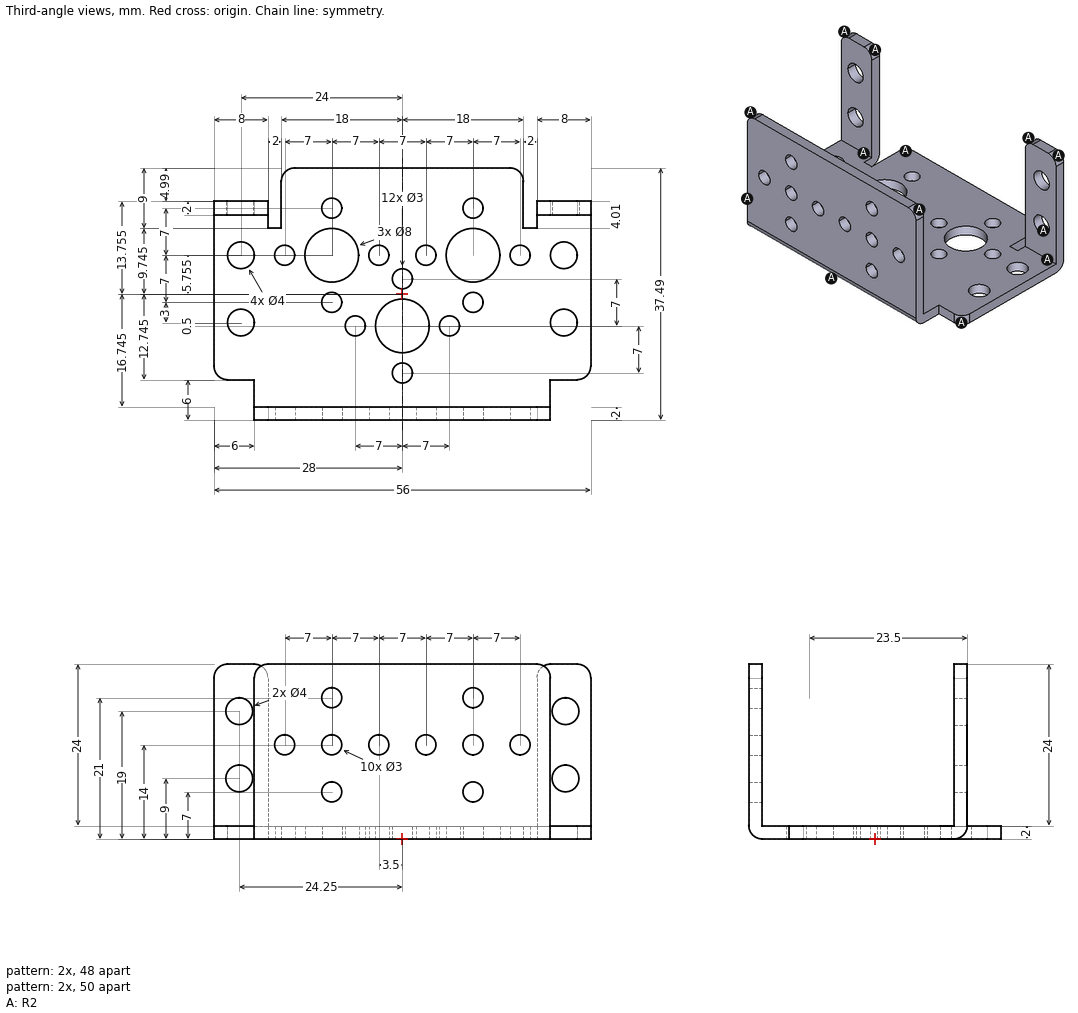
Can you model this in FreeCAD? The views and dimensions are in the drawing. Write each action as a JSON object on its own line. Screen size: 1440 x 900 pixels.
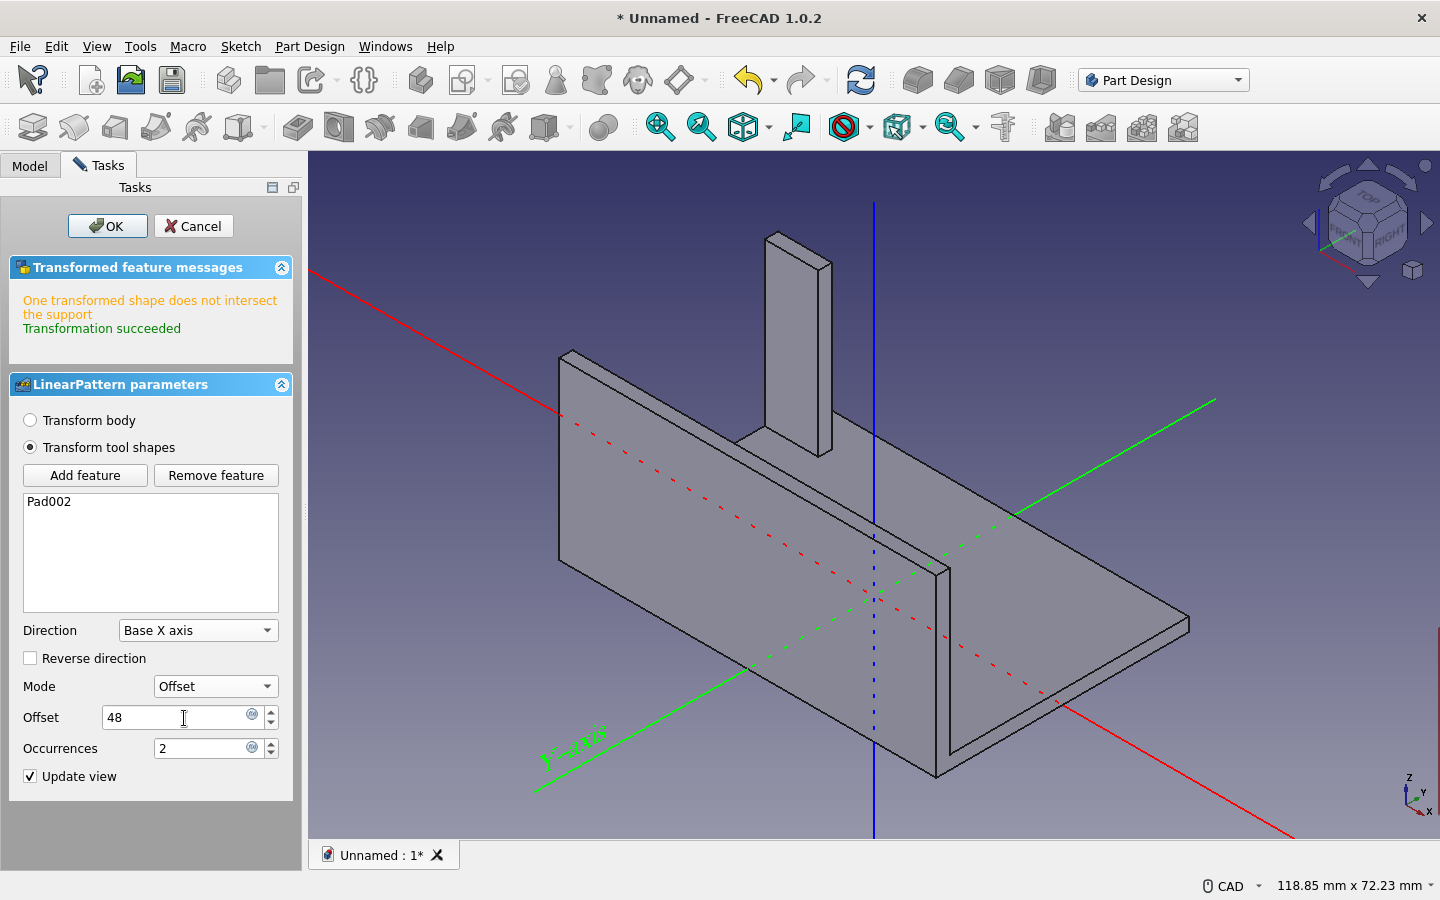
{"action": "triple_click", "coordinate": [210, 748]}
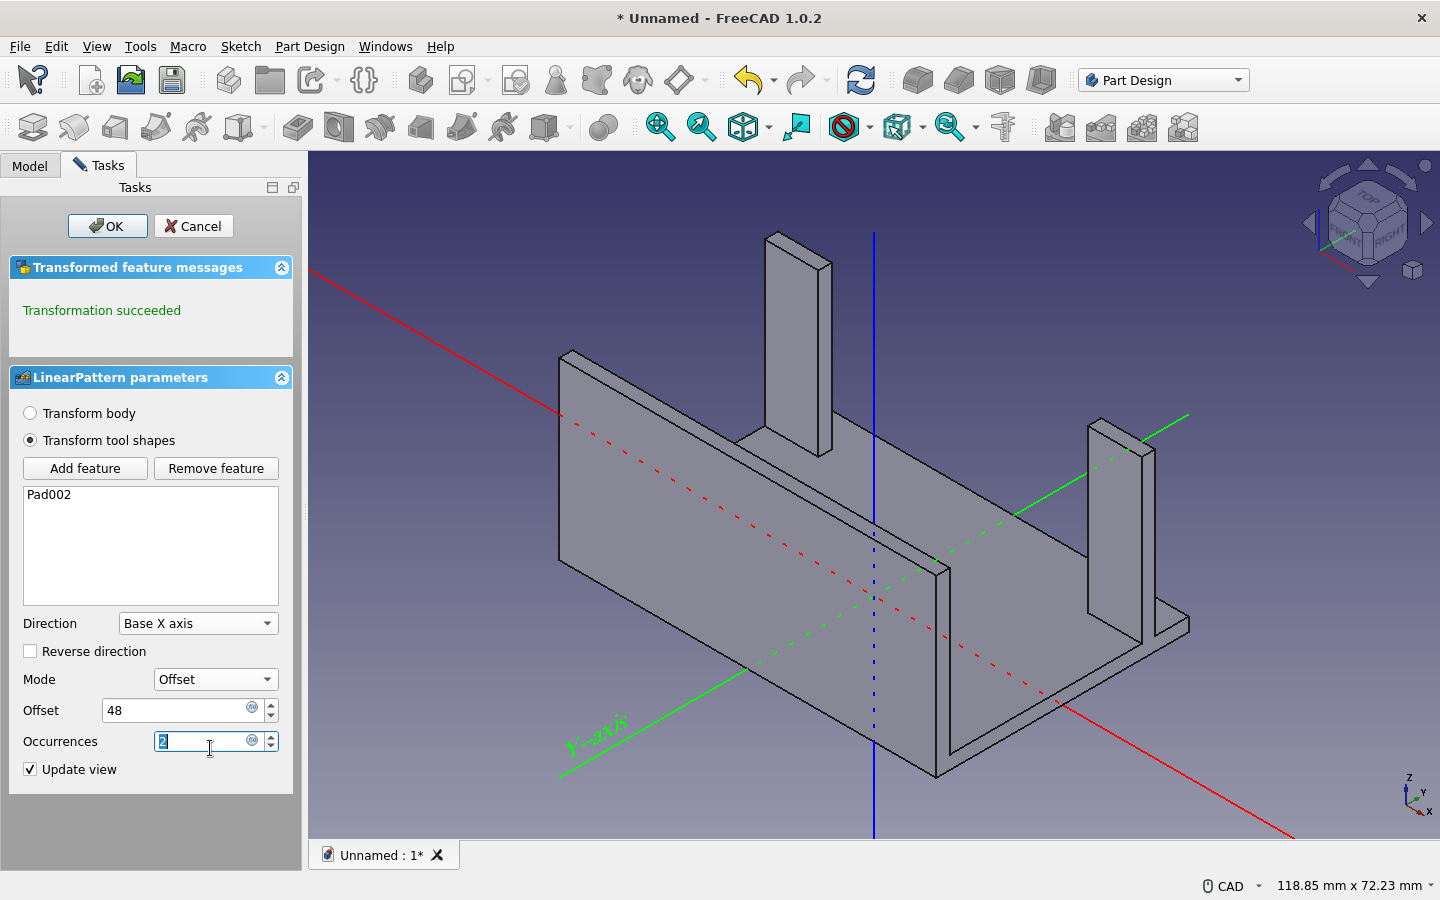
{"action": "type", "text": "2"}
{"action": "key", "text": "Tab"}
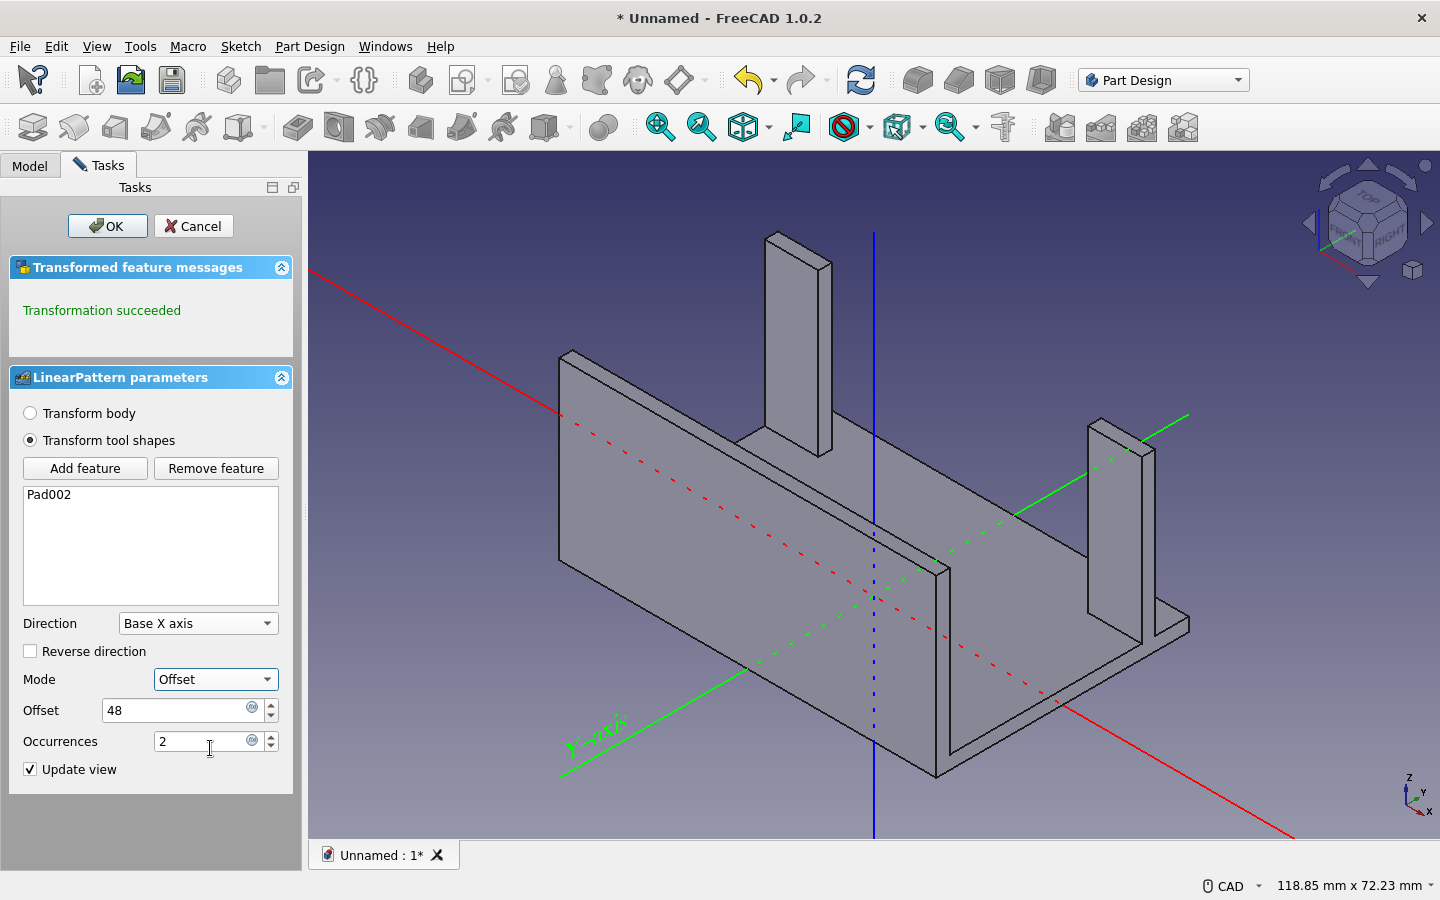
{"action": "left_click", "coordinate": [108, 226]}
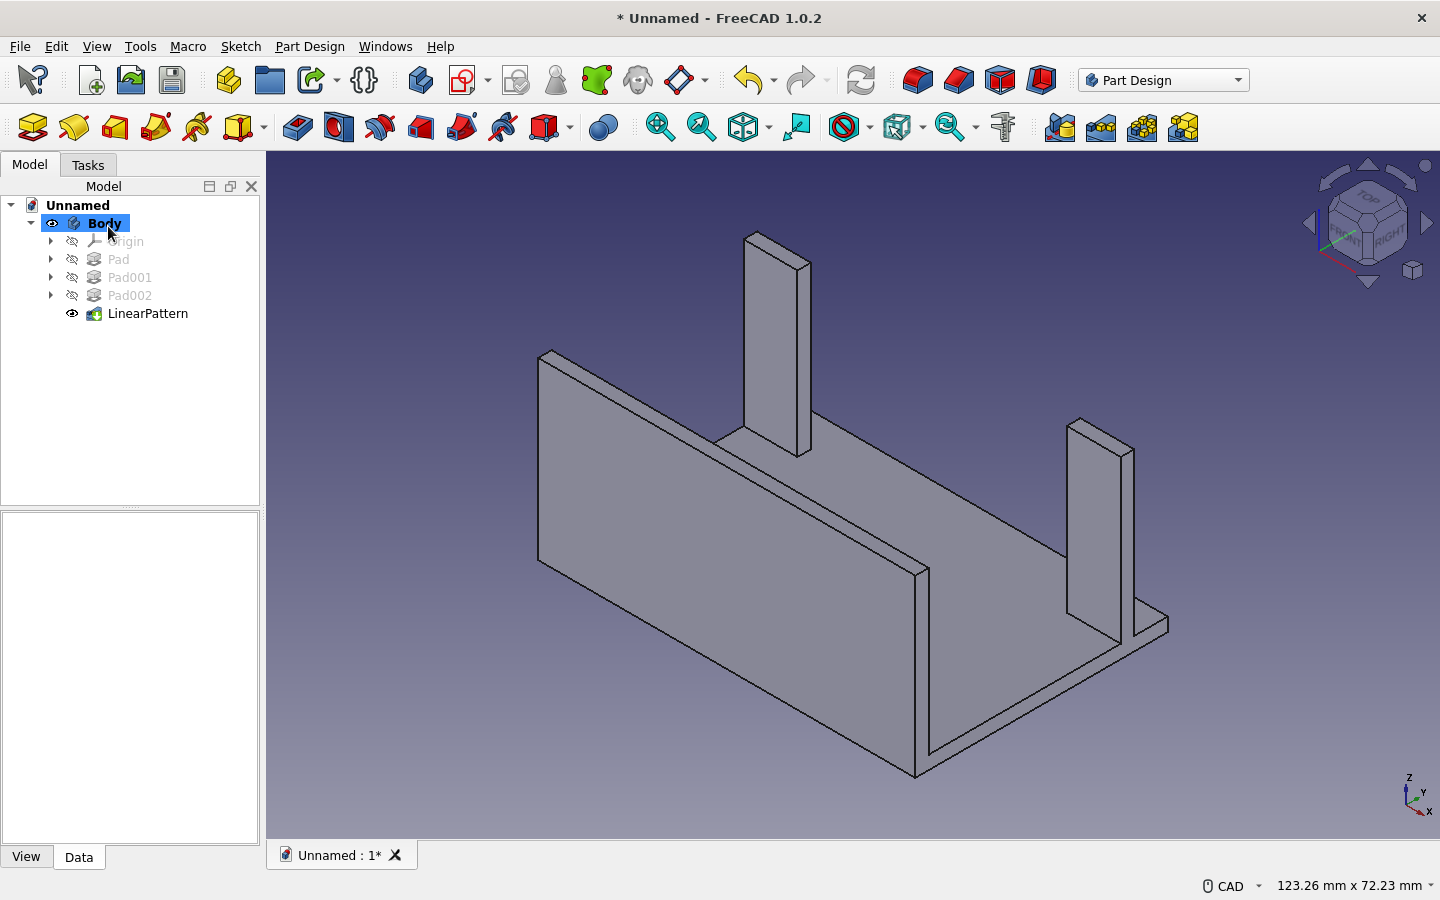
{"action": "left_click", "coordinate": [948, 587]}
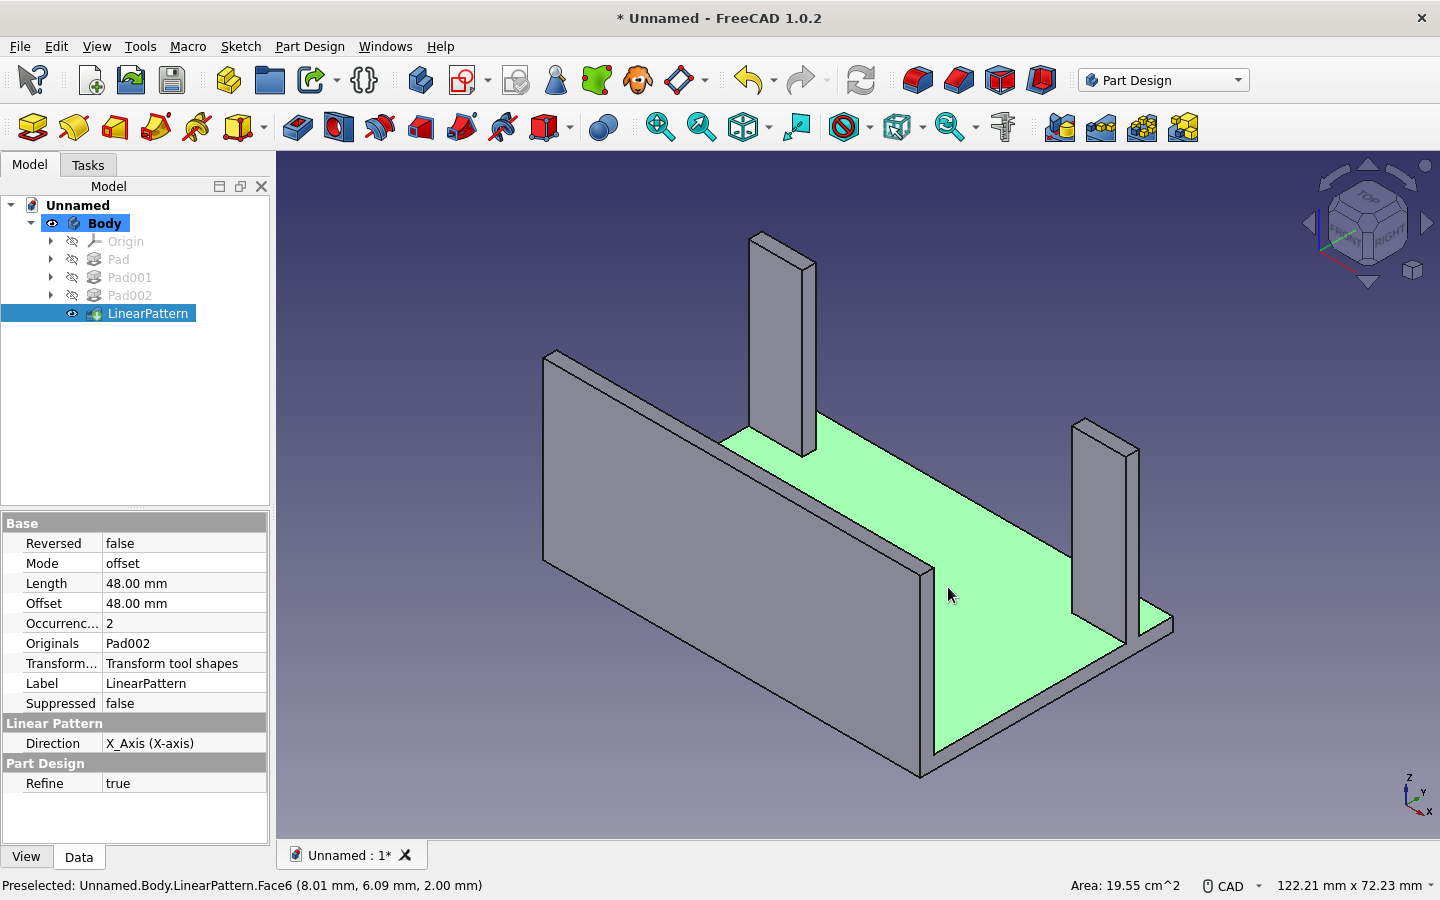
{"action": "left_click", "coordinate": [462, 80]}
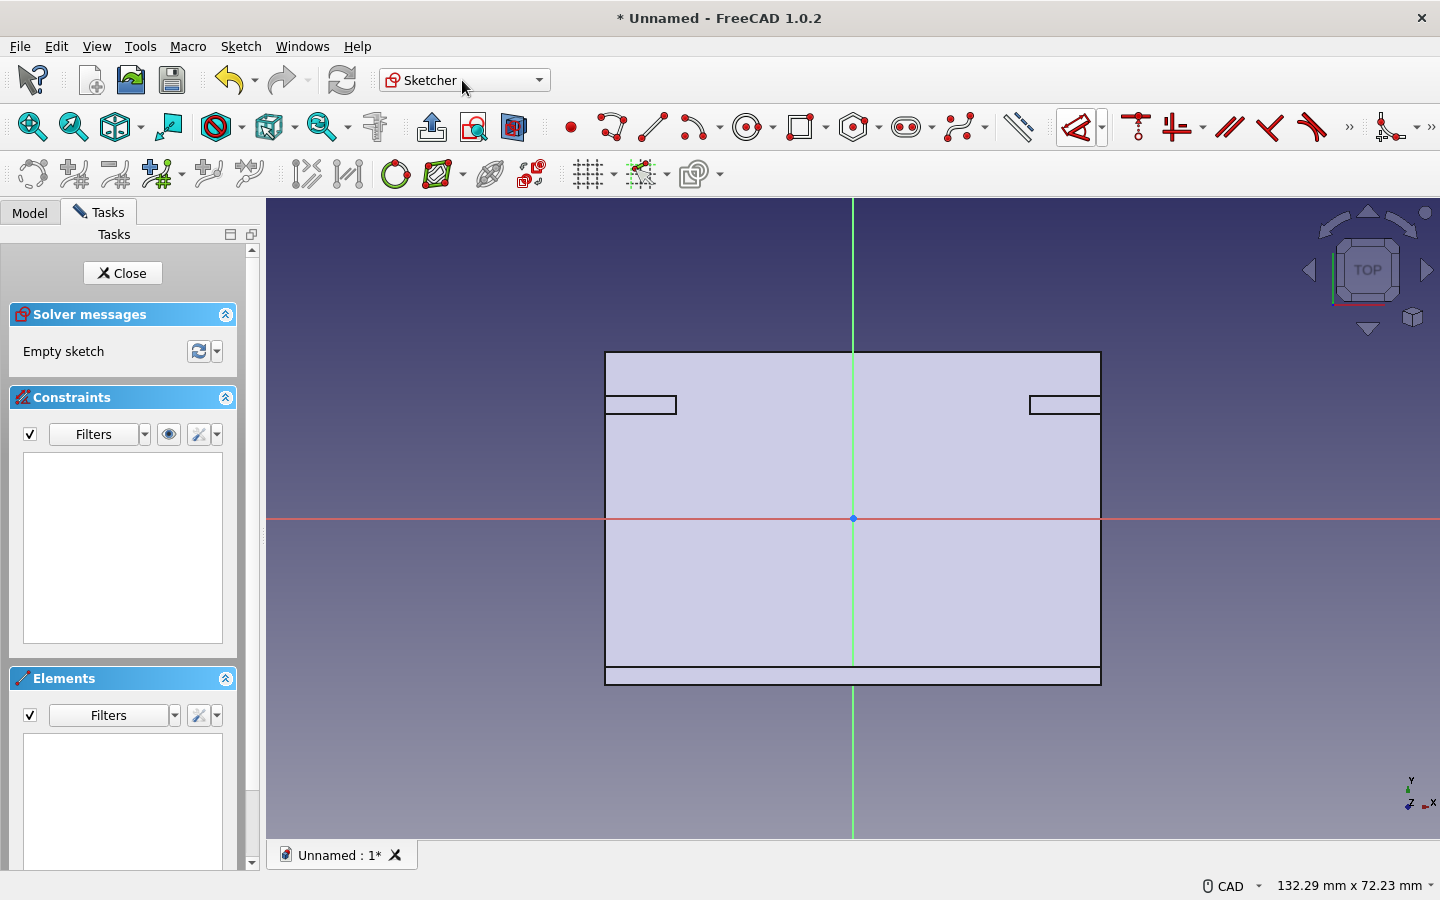
{"action": "scroll", "coordinate": [607, 680], "scroll_direction": "up", "scroll_amount": 10}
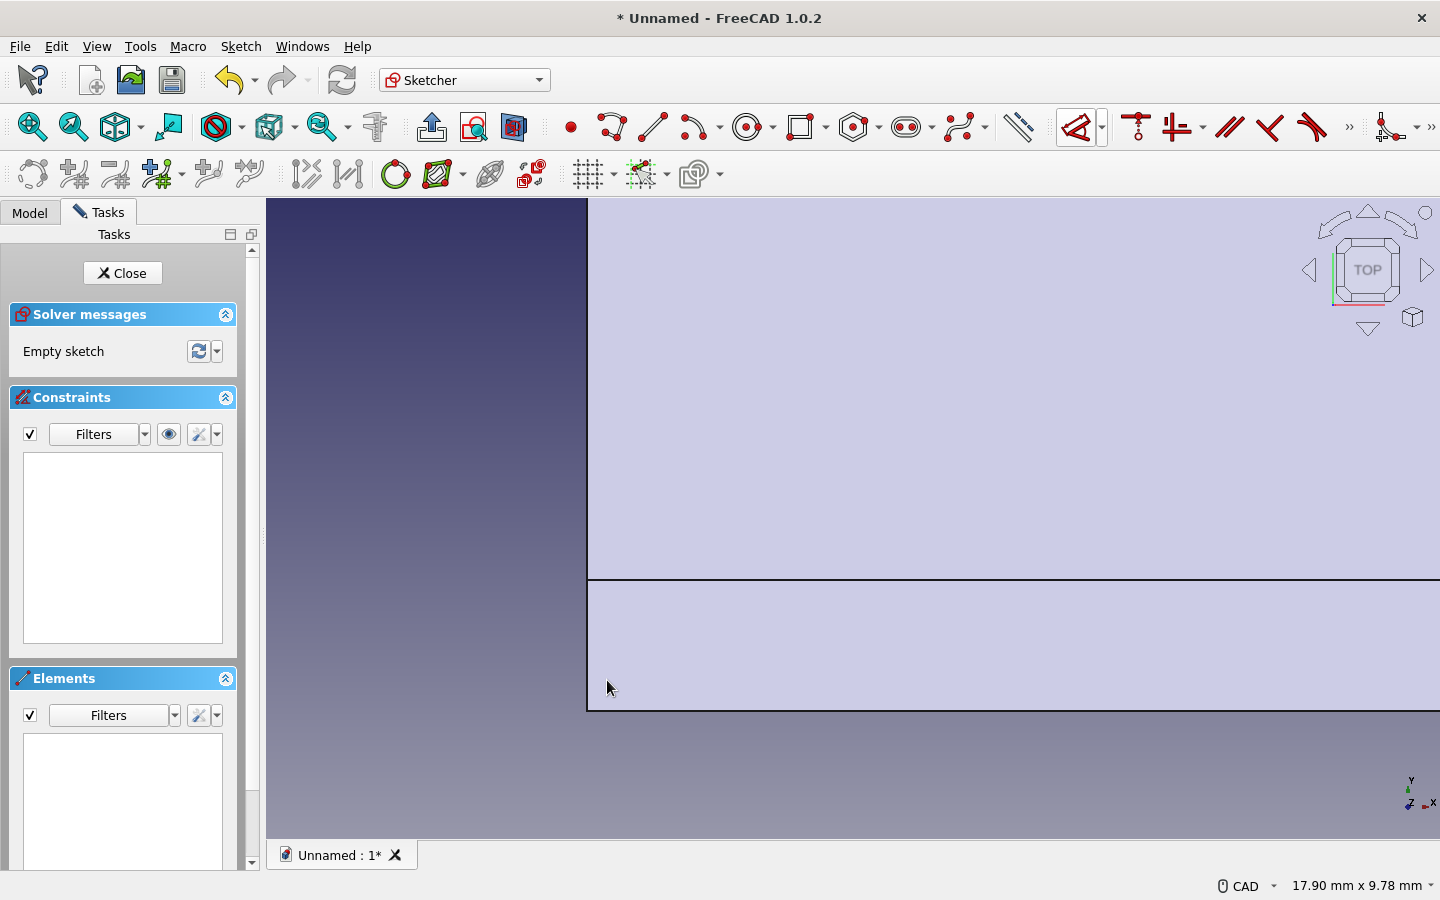
{"action": "key", "text": "g r"}